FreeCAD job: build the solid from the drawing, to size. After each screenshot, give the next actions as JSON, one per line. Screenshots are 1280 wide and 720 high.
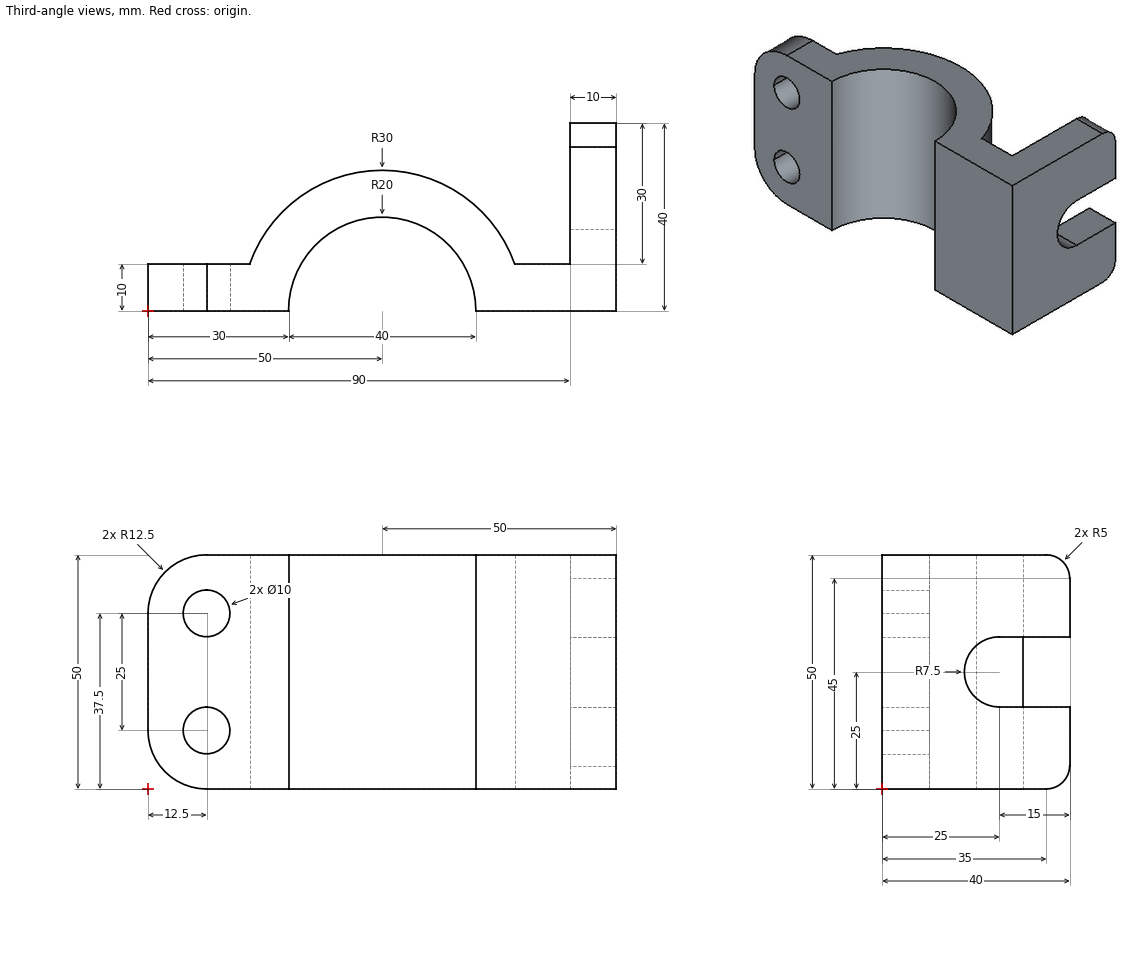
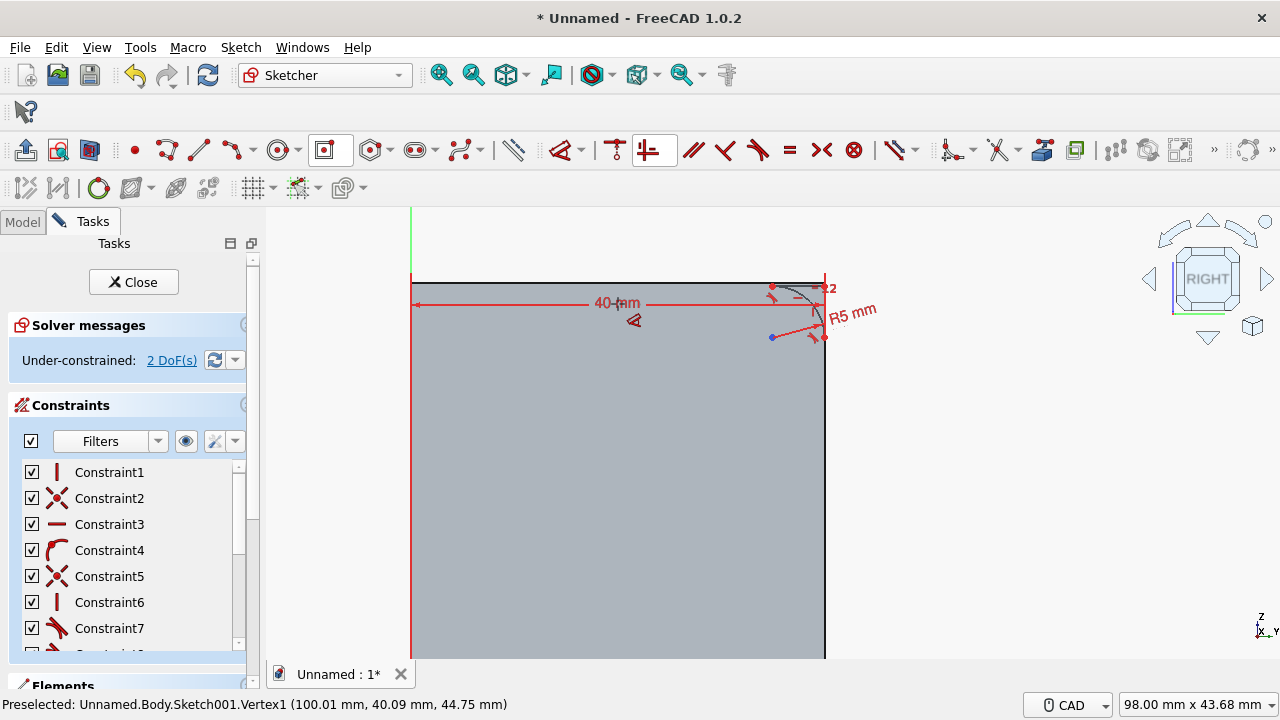
{"action": "left_click", "coordinate": [825, 338]}
{"action": "left_click", "coordinate": [859, 484]}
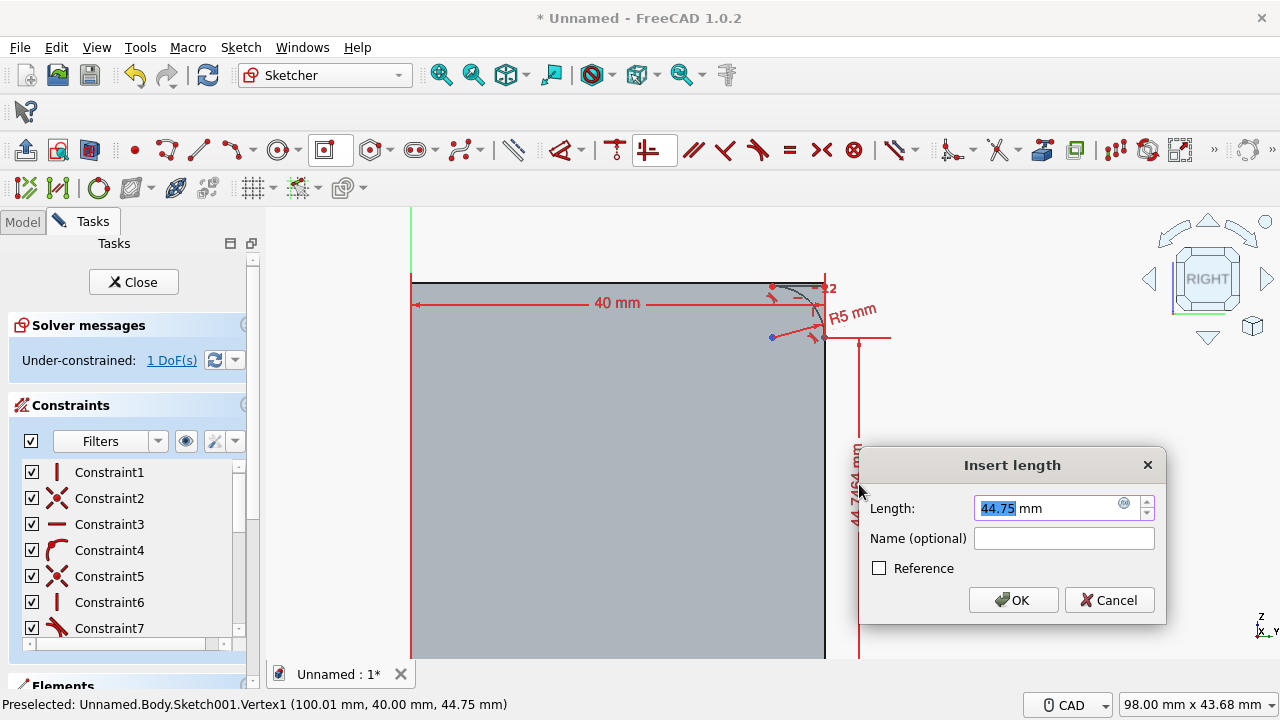
{"action": "type", "text": "45"}
{"action": "key", "text": "Return"}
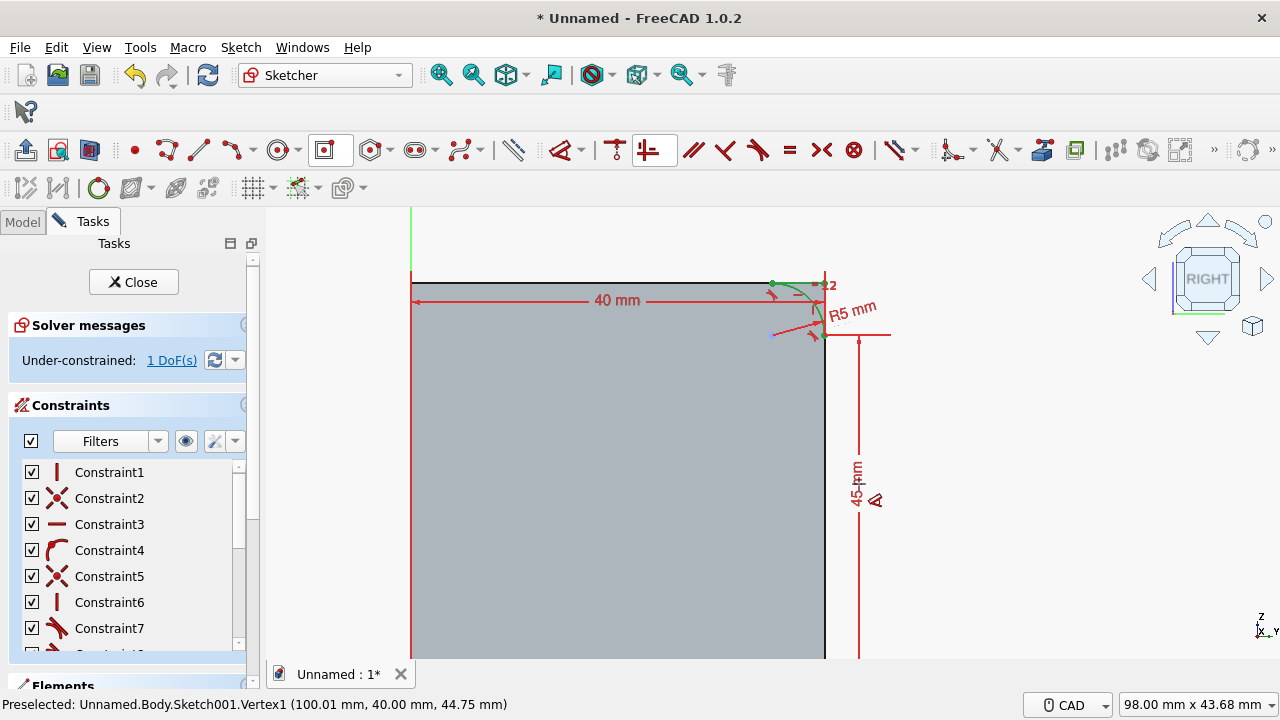
{"action": "scroll", "coordinate": [810, 300], "scroll_direction": "down", "scroll_amount": 3}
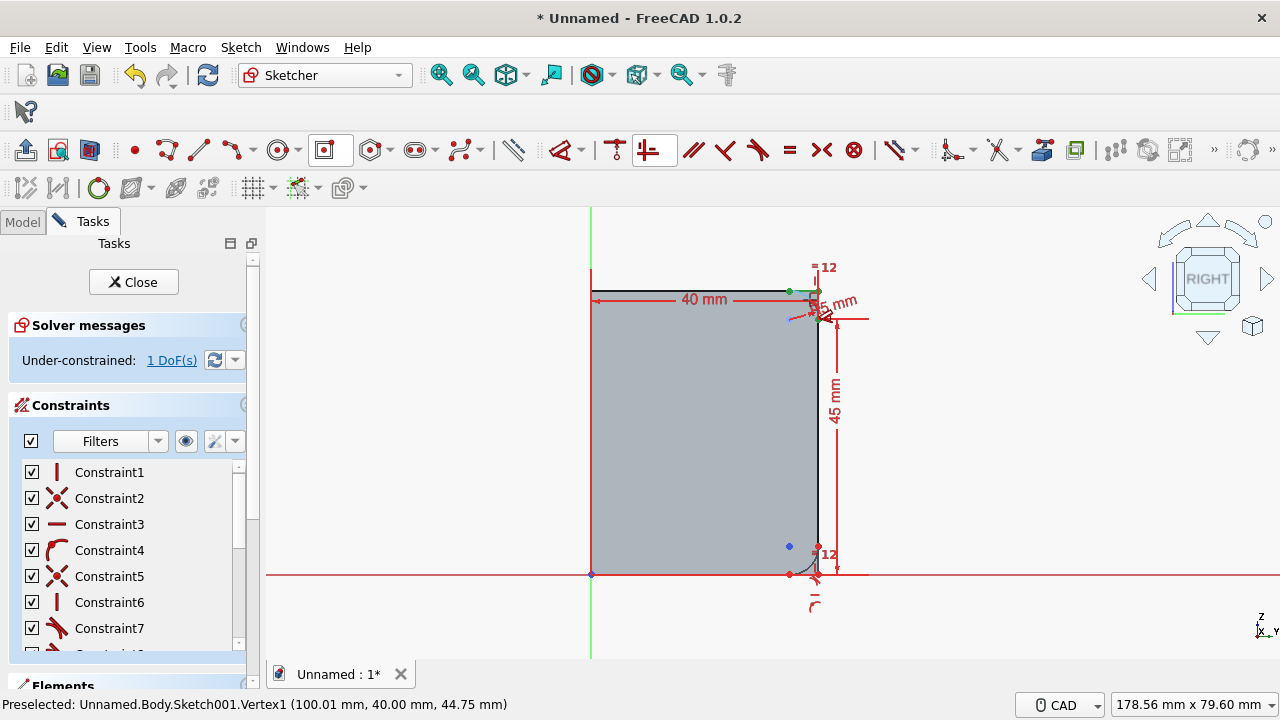
{"action": "left_click", "coordinate": [790, 575]}
{"action": "left_click", "coordinate": [690, 609]}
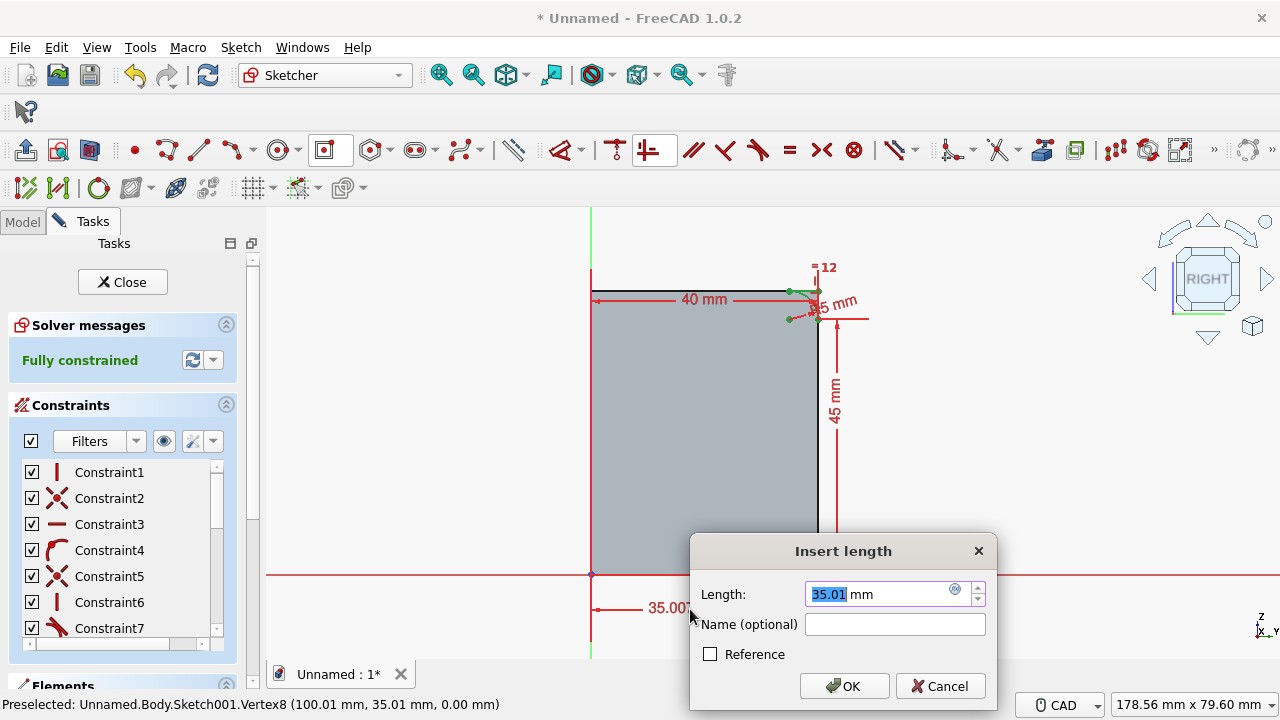
{"action": "type", "text": "35"}
{"action": "key", "text": "Return"}
{"action": "key", "text": "Escape"}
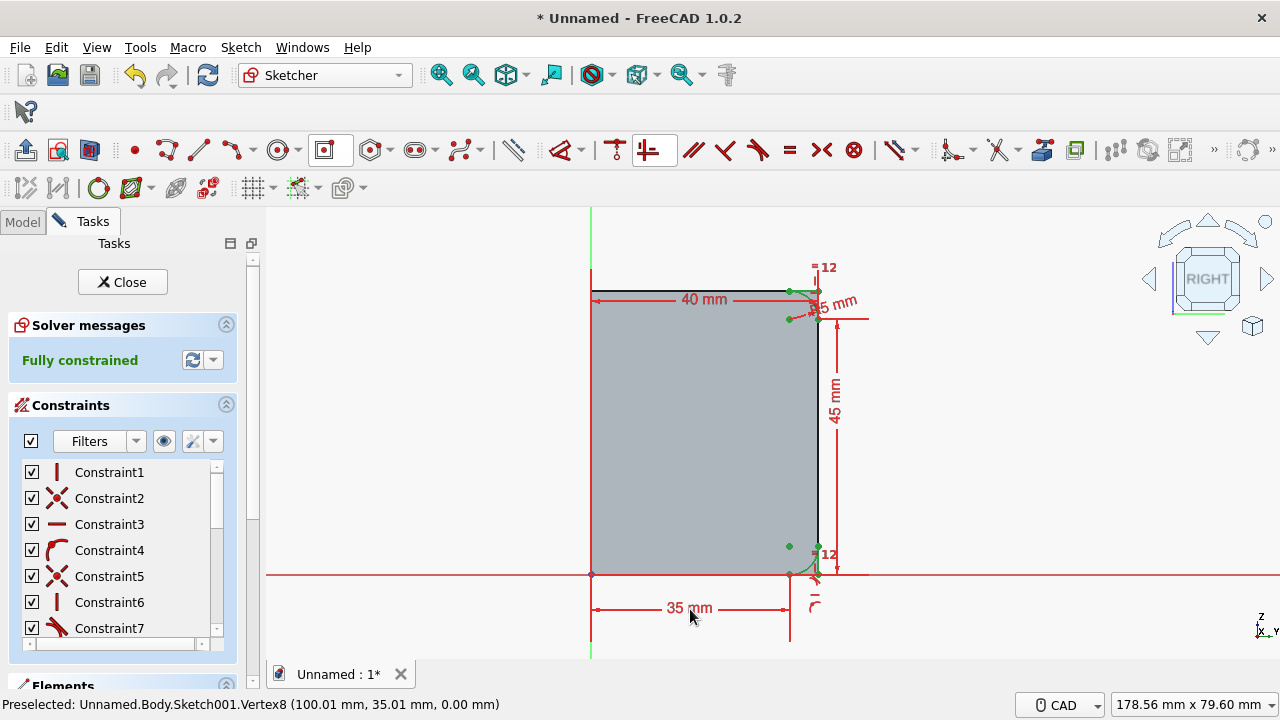
{"action": "left_click", "coordinate": [123, 282]}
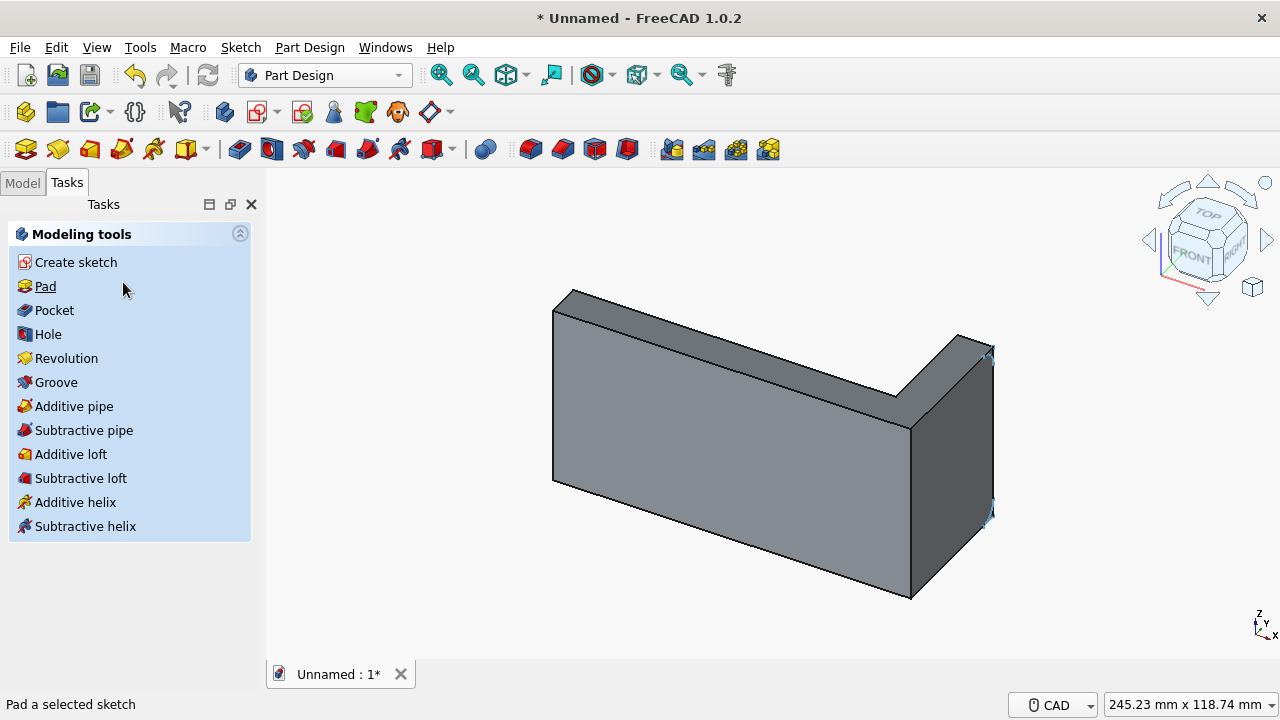
{"action": "left_click", "coordinate": [240, 150]}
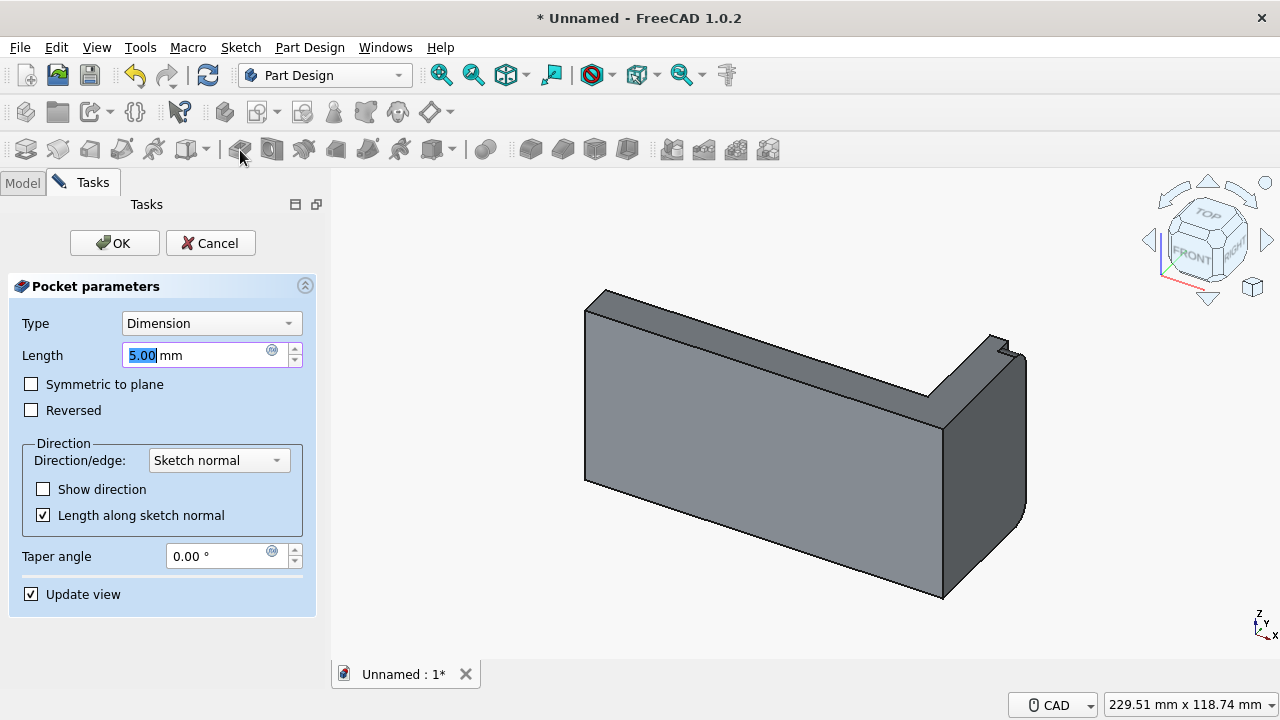
{"action": "type", "text": "50"}
{"action": "key", "text": "Tab"}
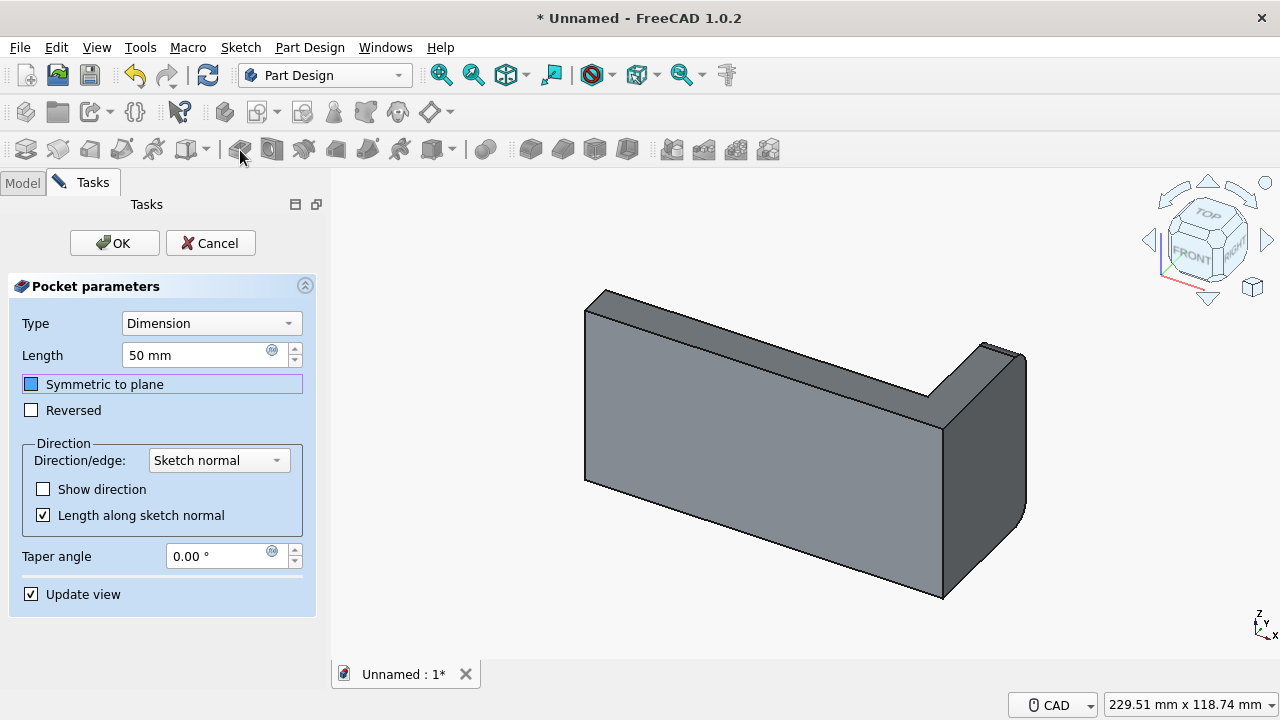
{"action": "left_click", "coordinate": [115, 243]}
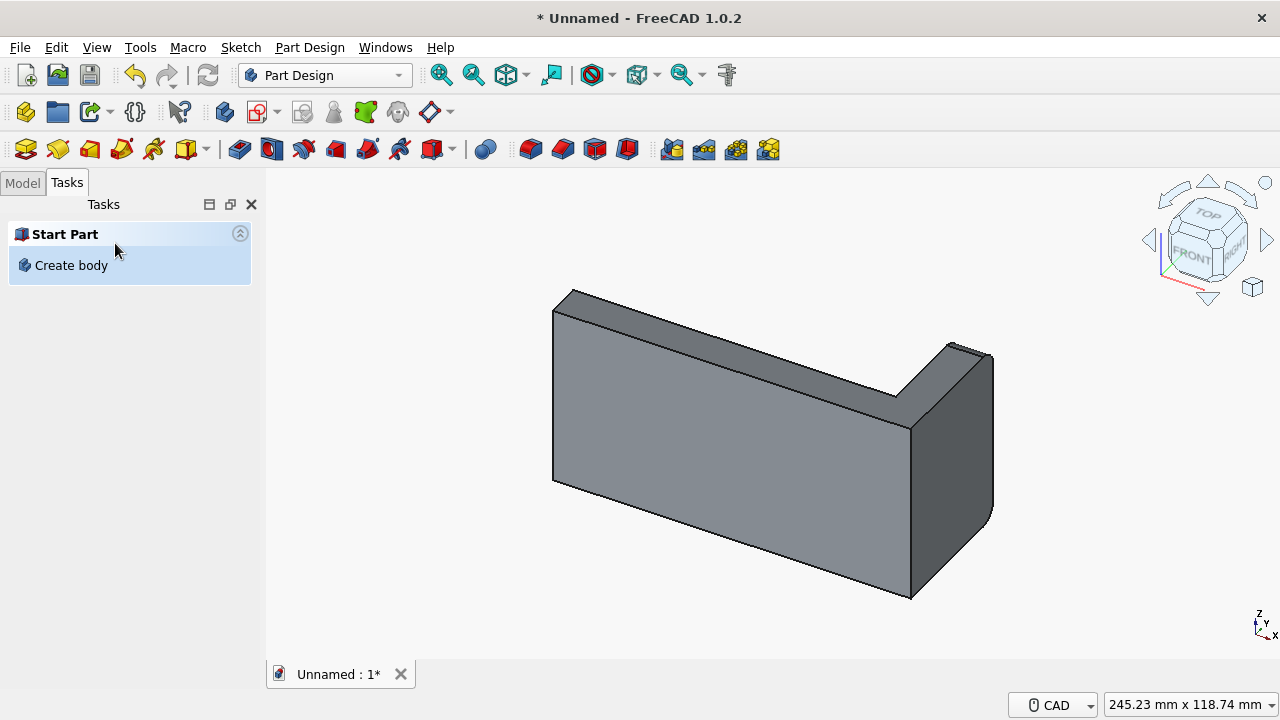
{"action": "left_click", "coordinate": [952, 472]}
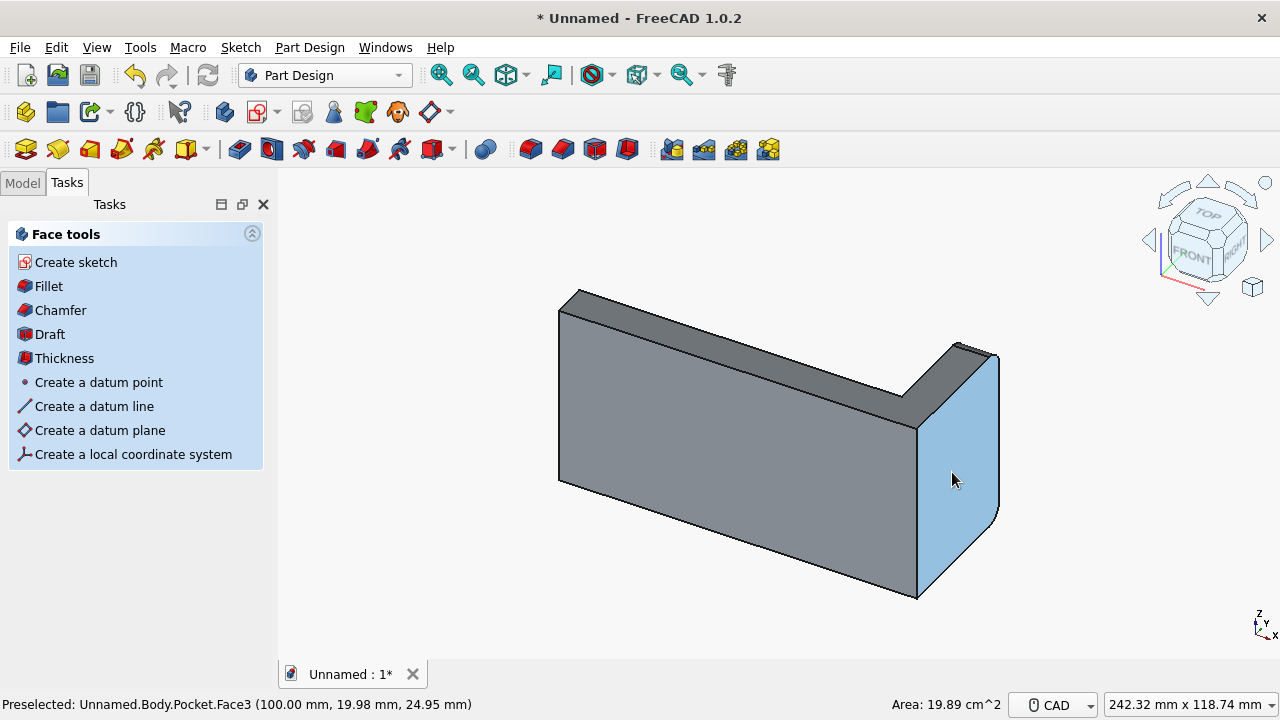
{"action": "left_click", "coordinate": [258, 112]}